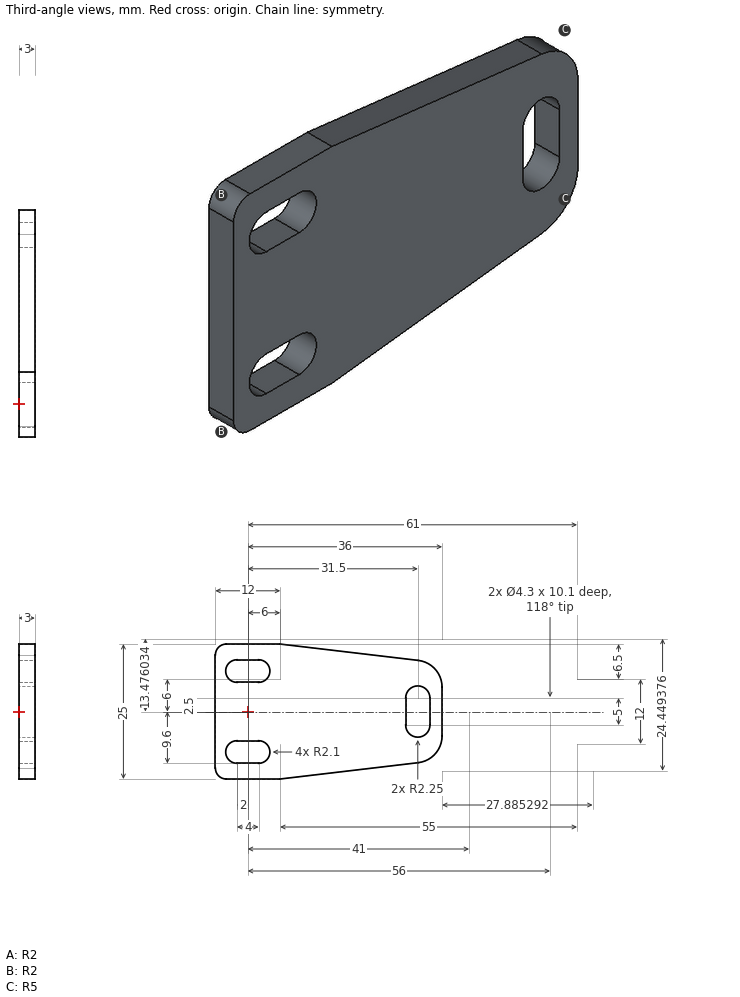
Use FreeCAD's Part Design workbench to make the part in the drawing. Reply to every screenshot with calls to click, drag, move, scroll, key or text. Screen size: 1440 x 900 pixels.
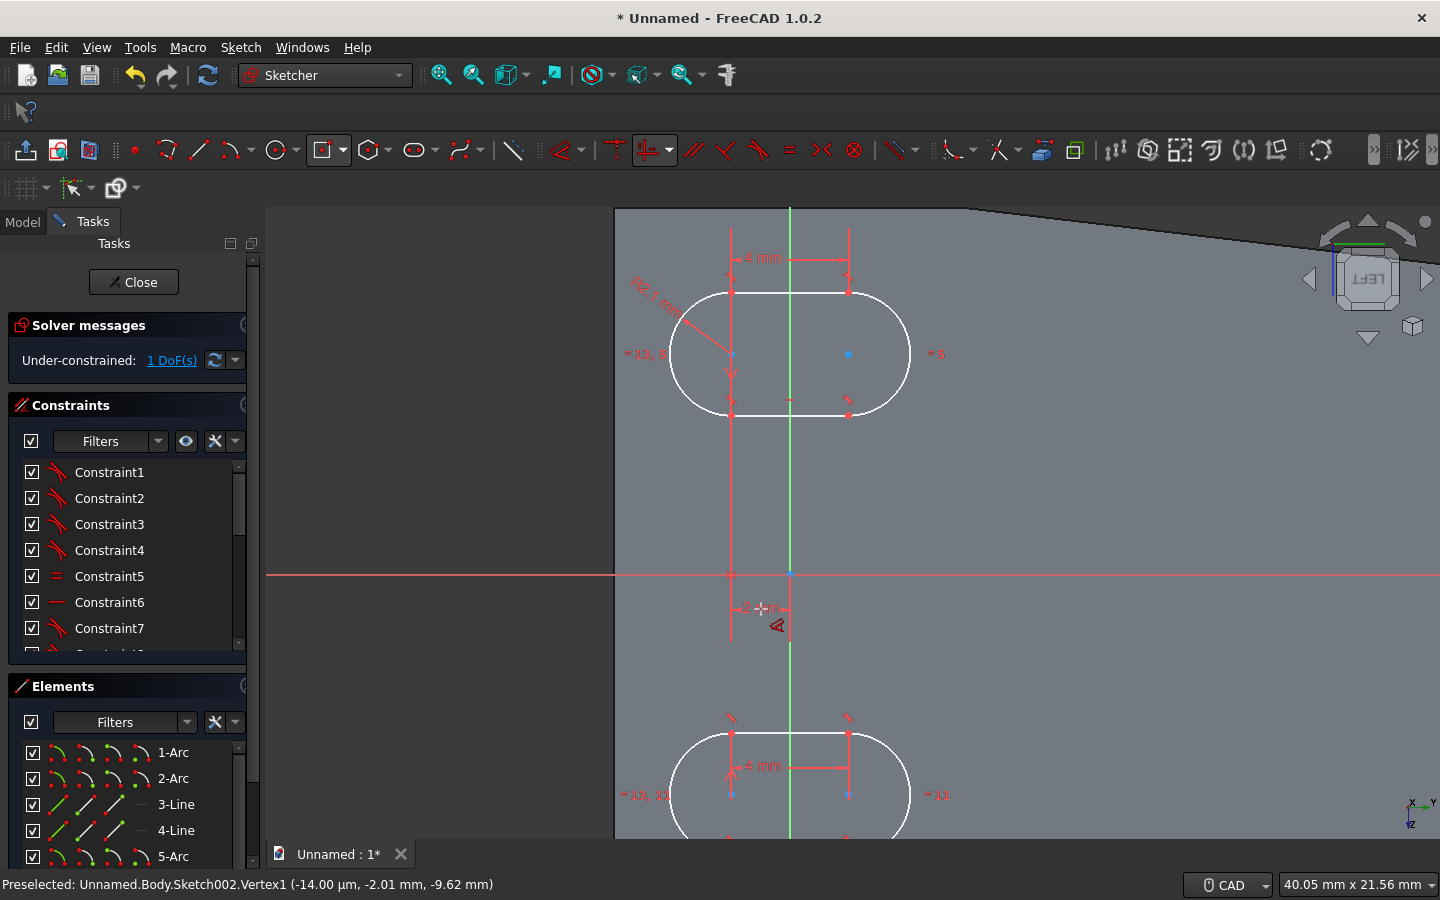
click(731, 293)
click(697, 434)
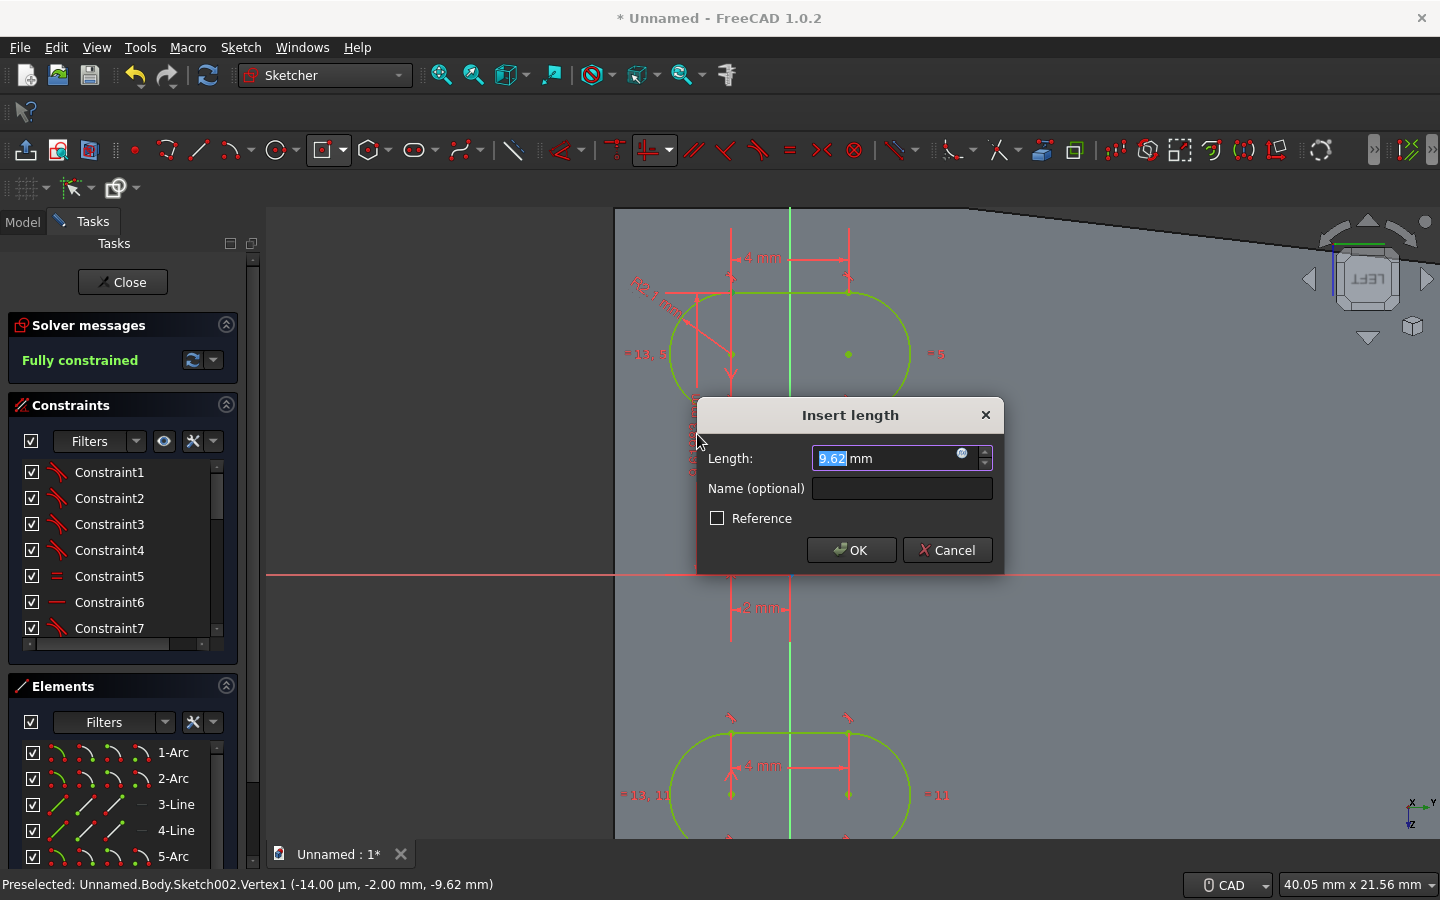
text(9.6)
key(Return)
key(Escape)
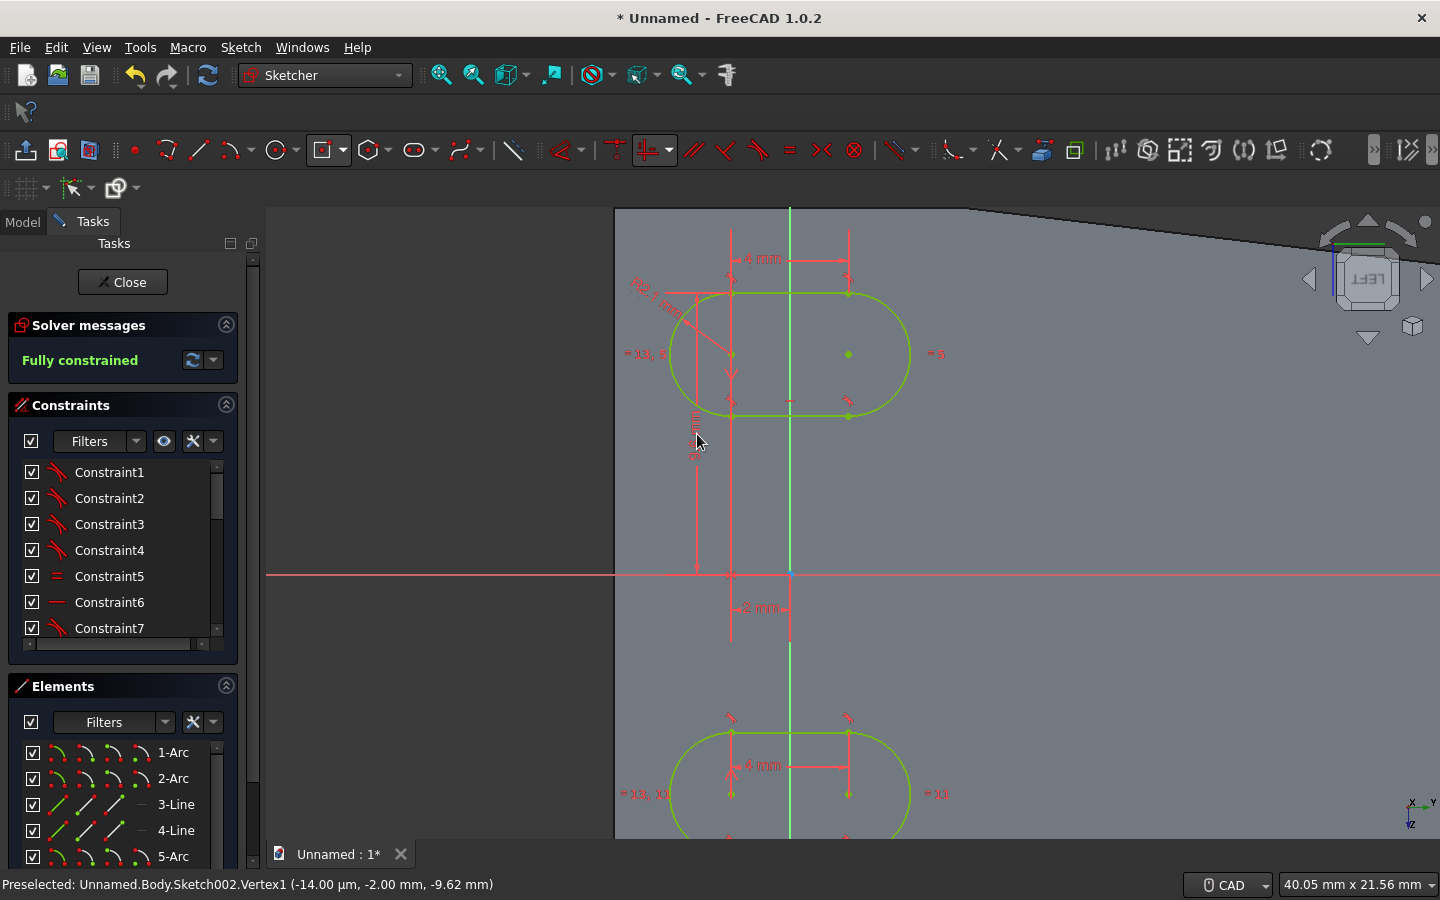
click(123, 282)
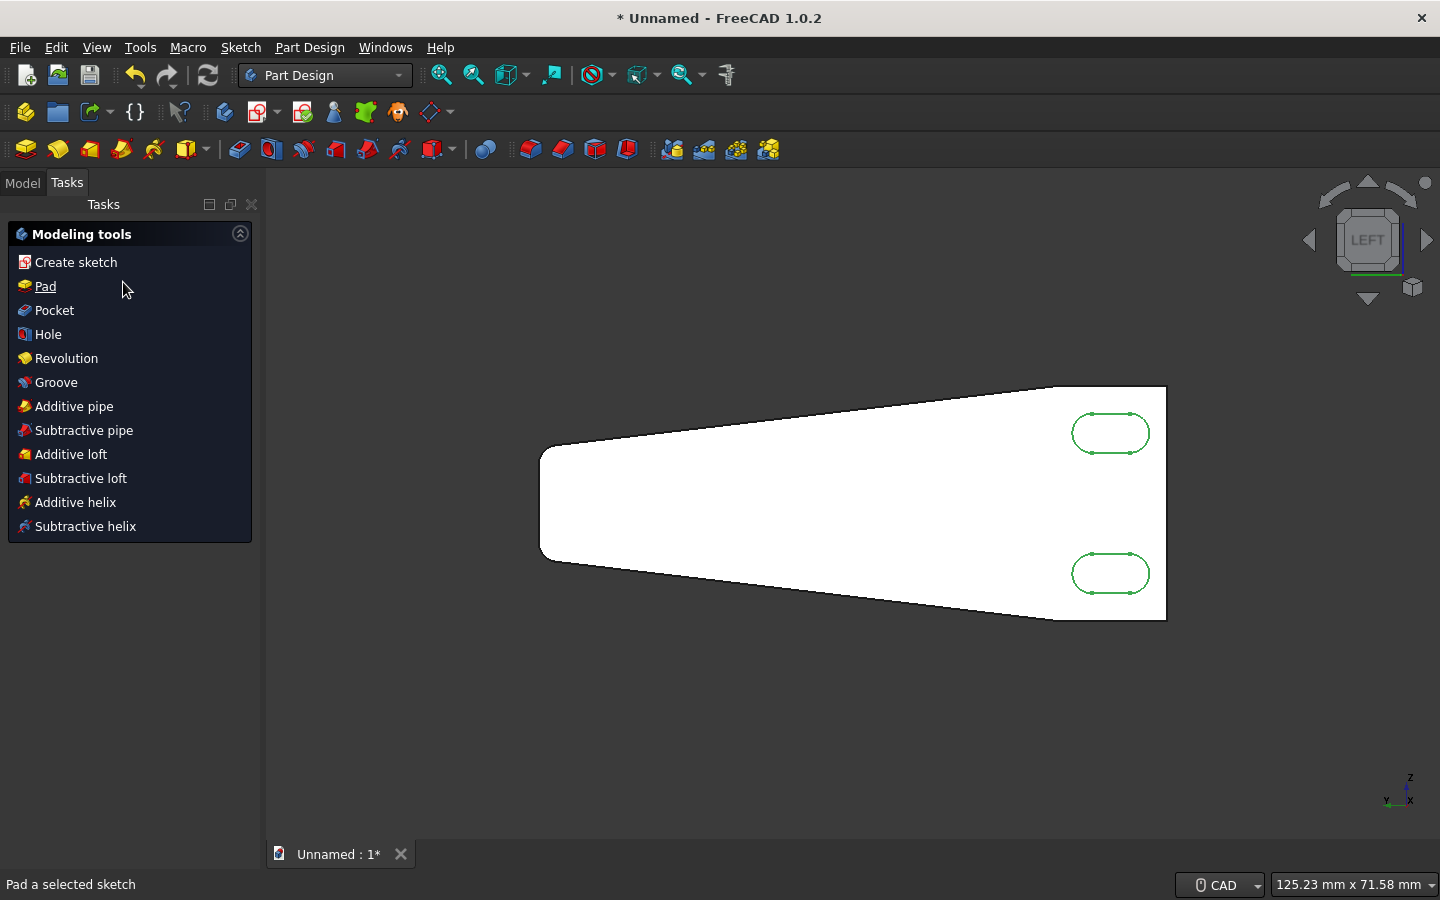
click(240, 150)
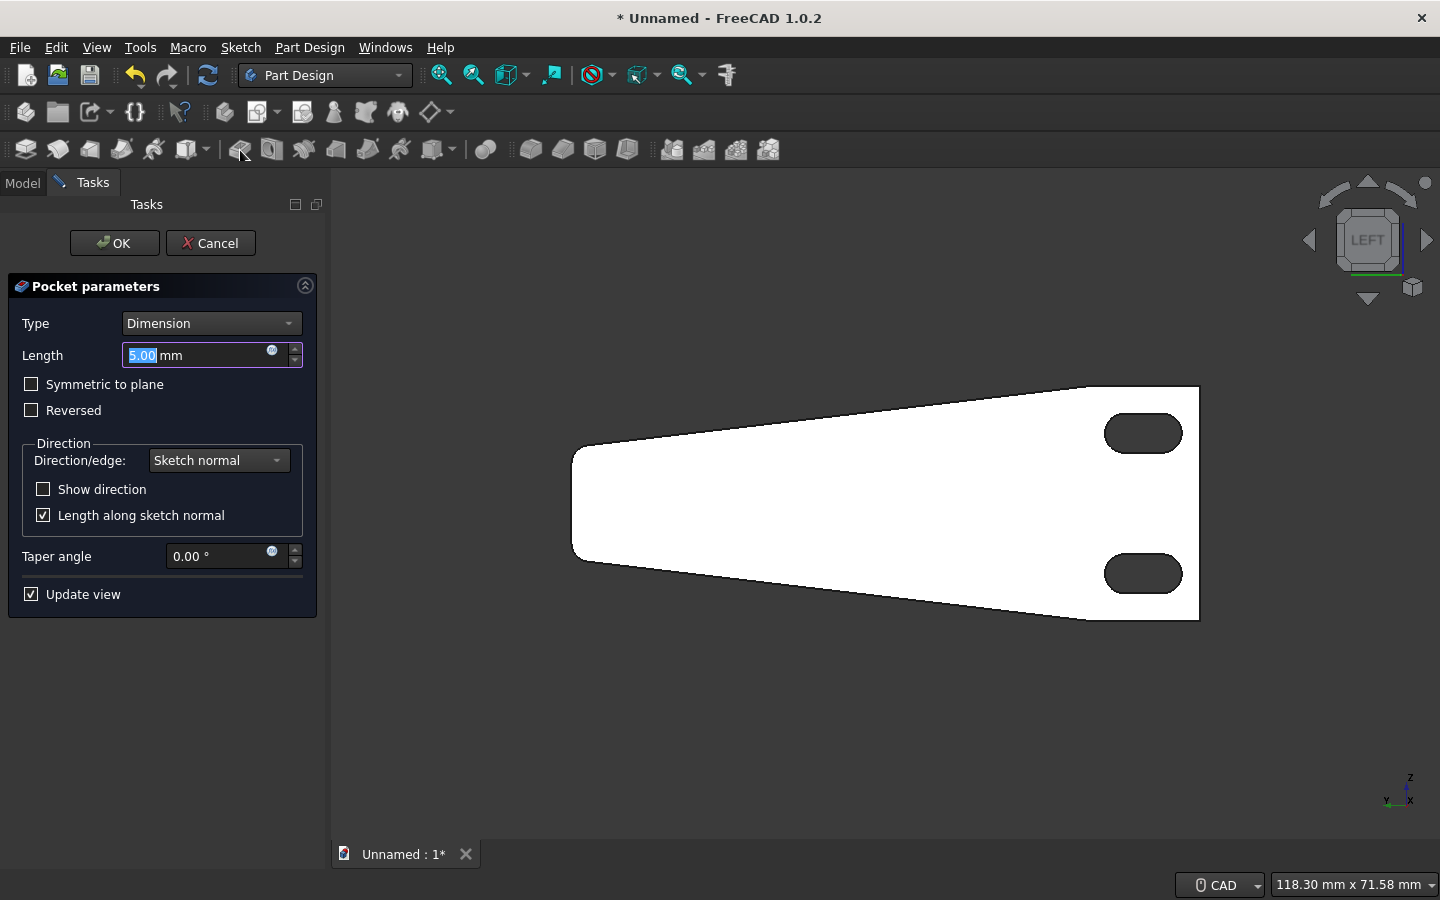
text(3)
key(Tab)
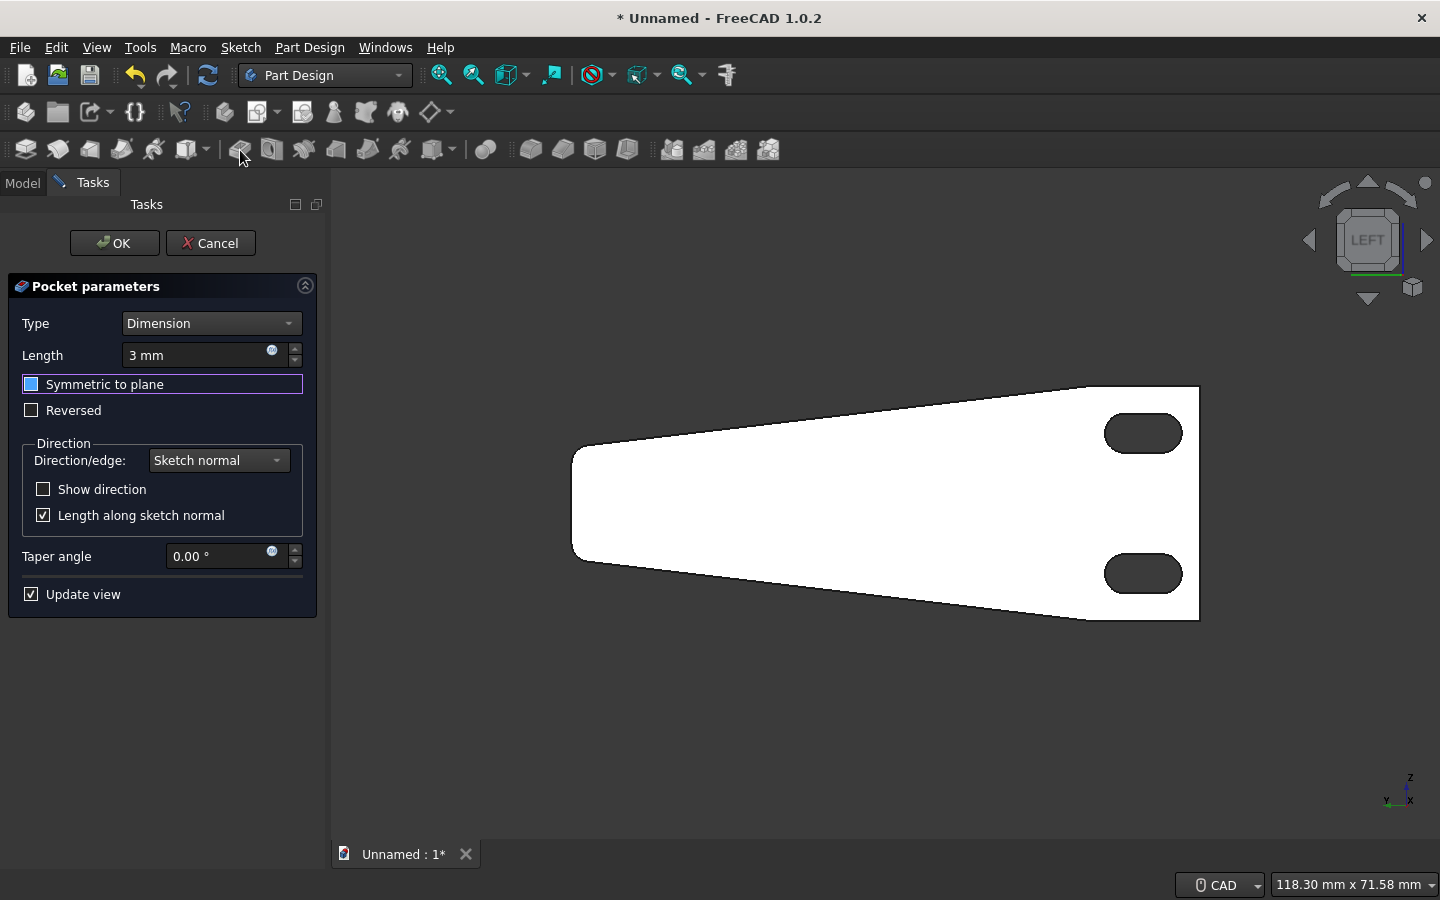
click(115, 243)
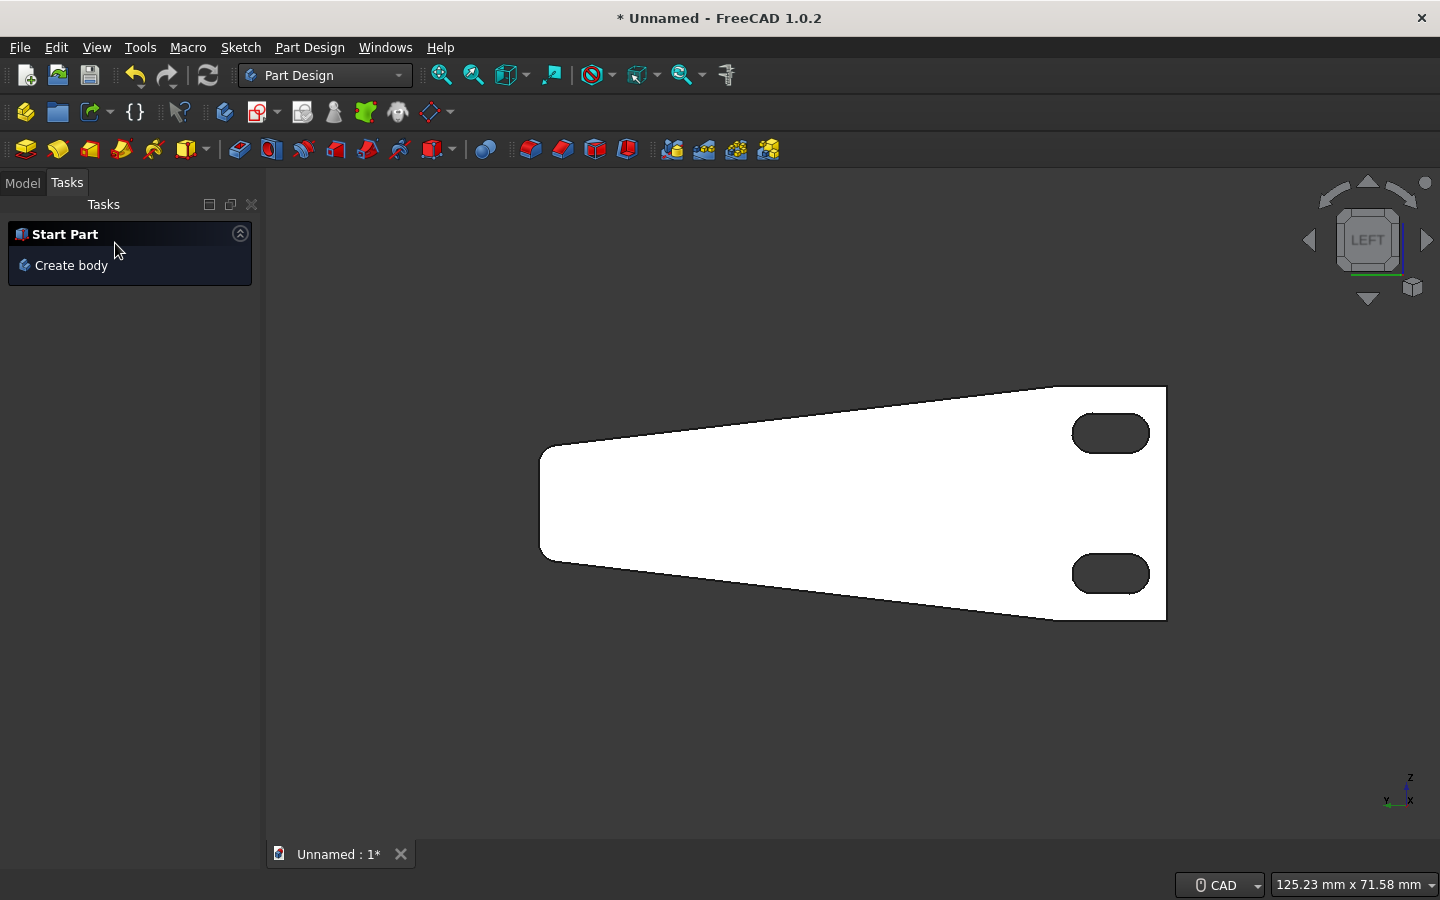
key(0)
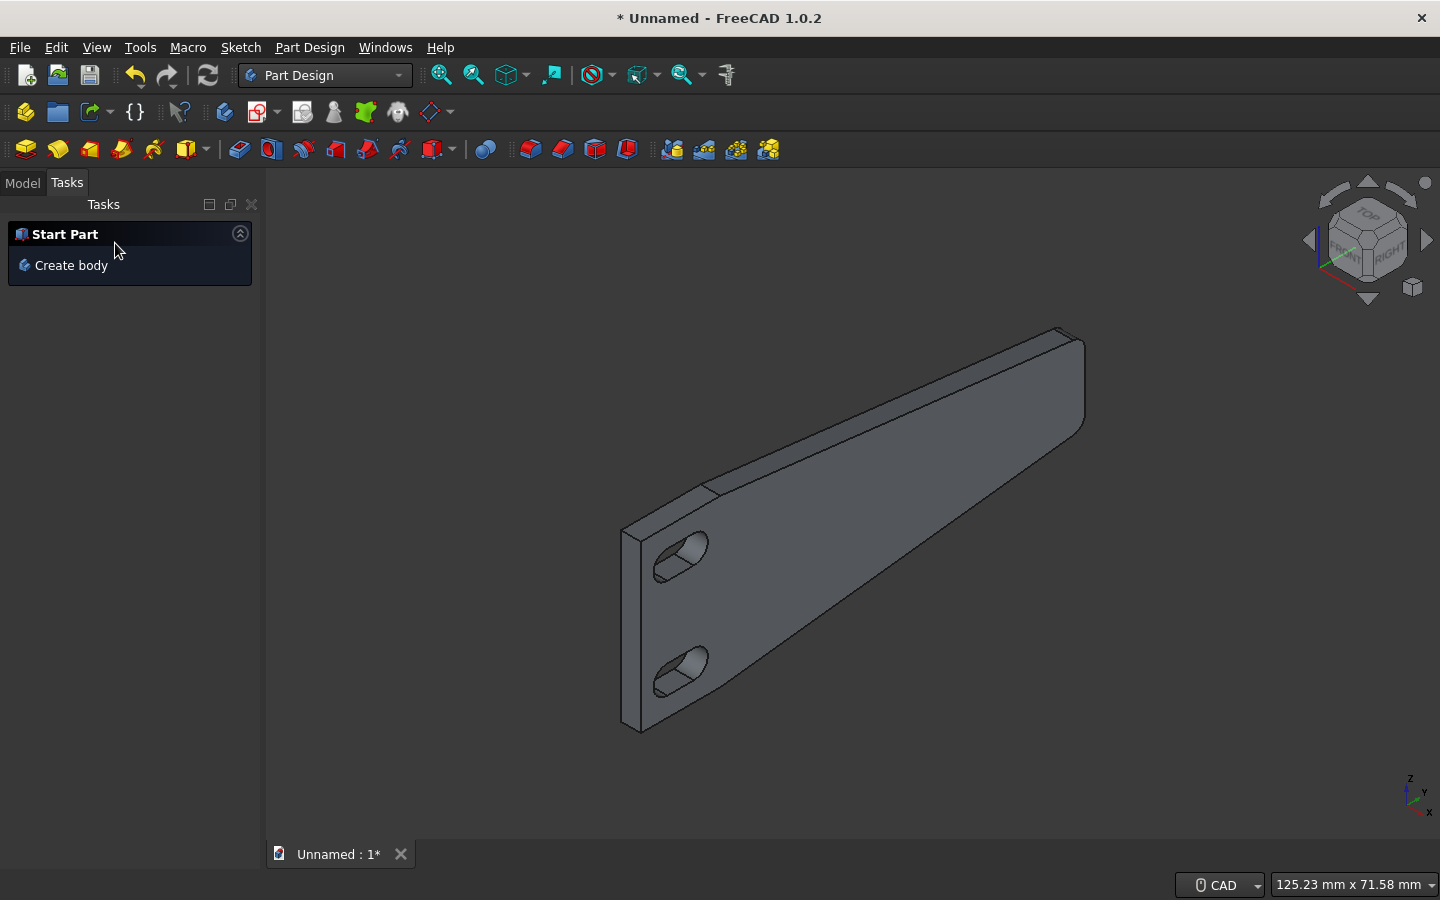
click(631, 535)